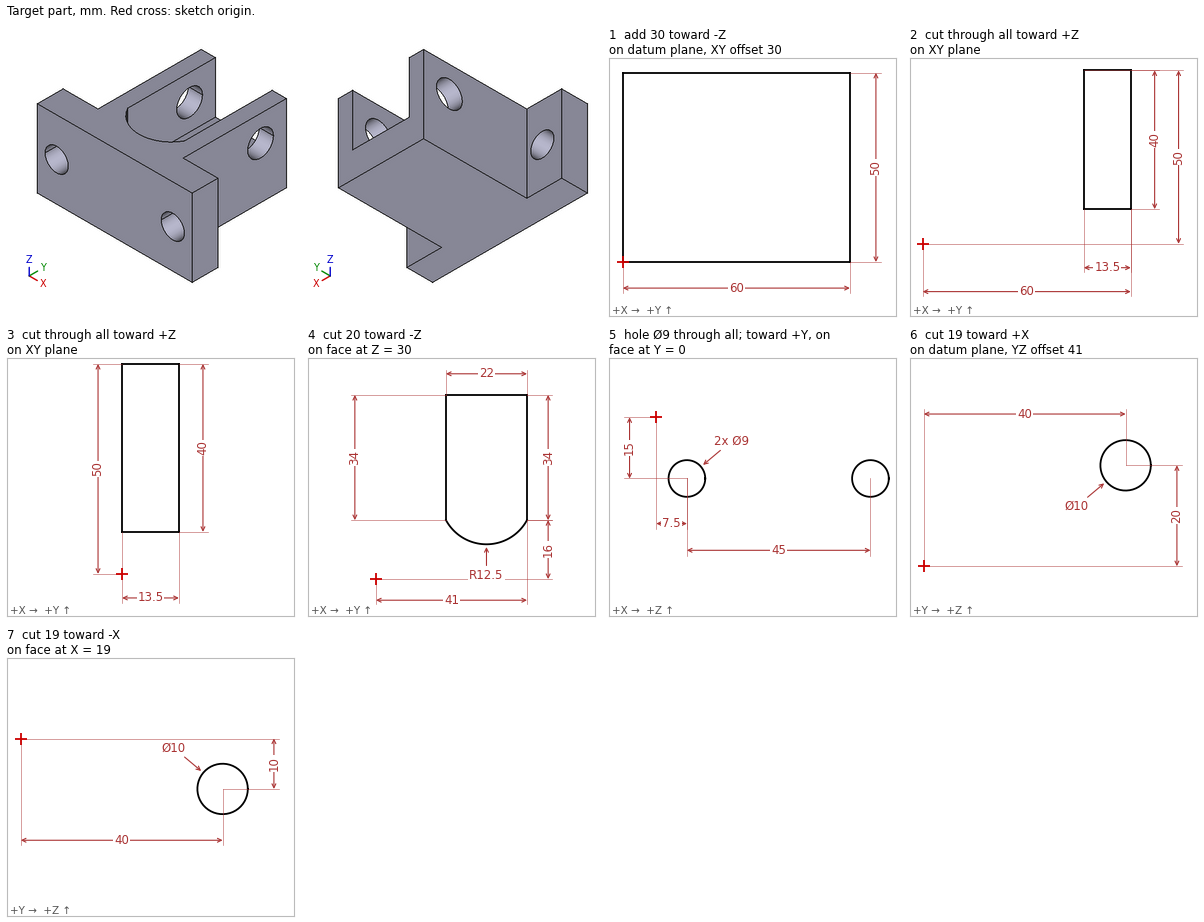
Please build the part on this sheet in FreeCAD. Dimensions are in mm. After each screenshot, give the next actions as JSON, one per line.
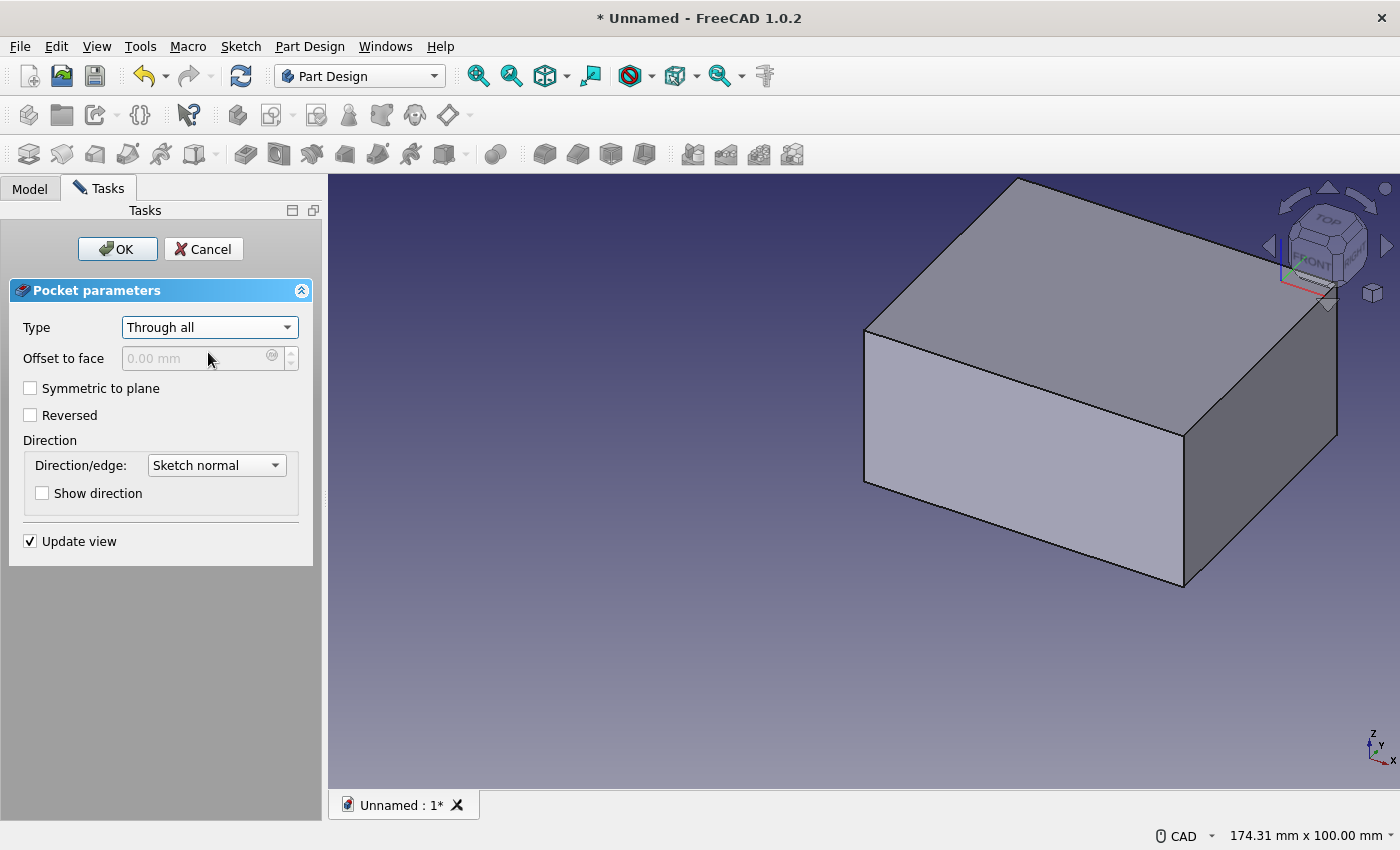
{"action": "left_click", "coordinate": [31, 415]}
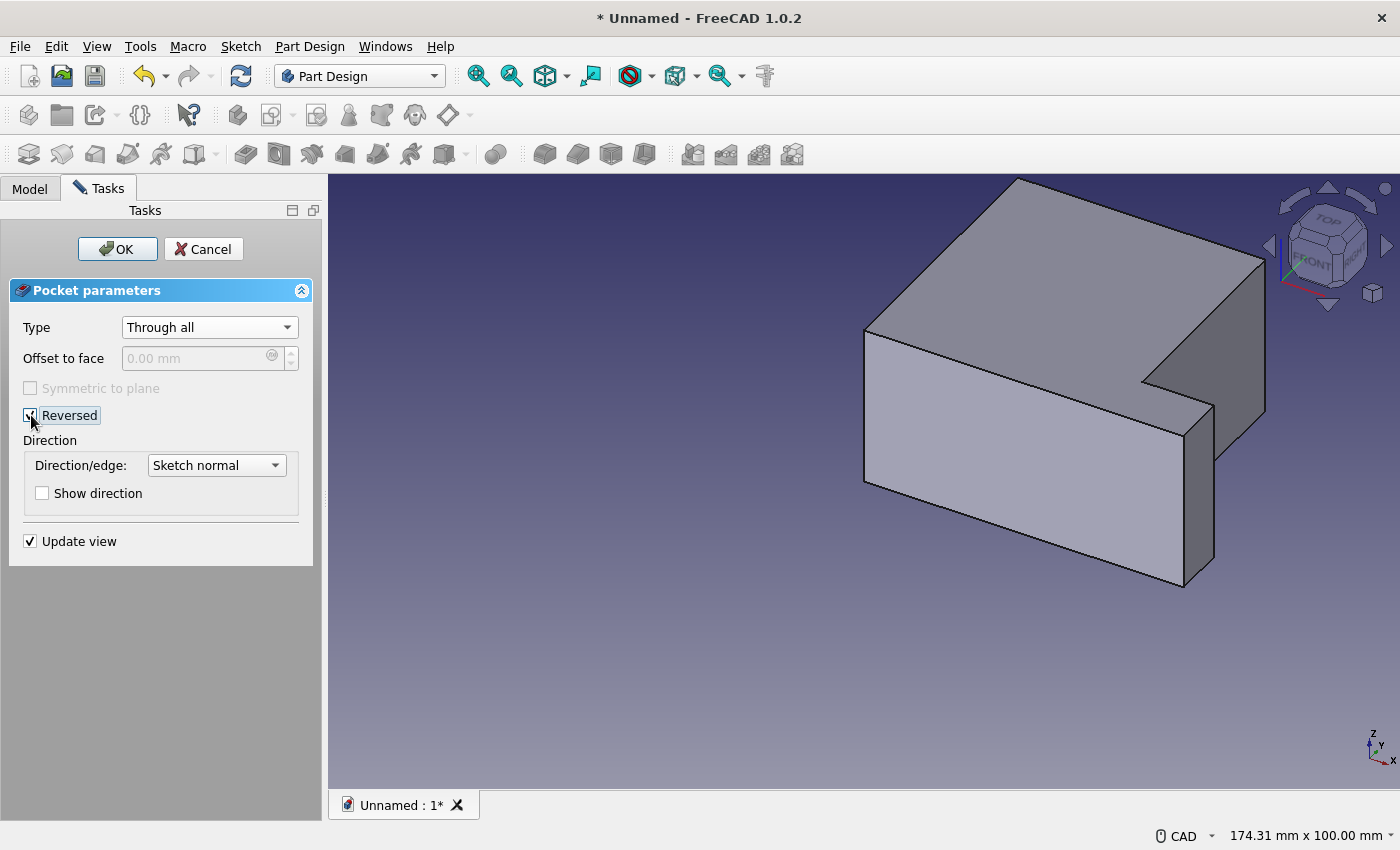
{"action": "left_click", "coordinate": [118, 249]}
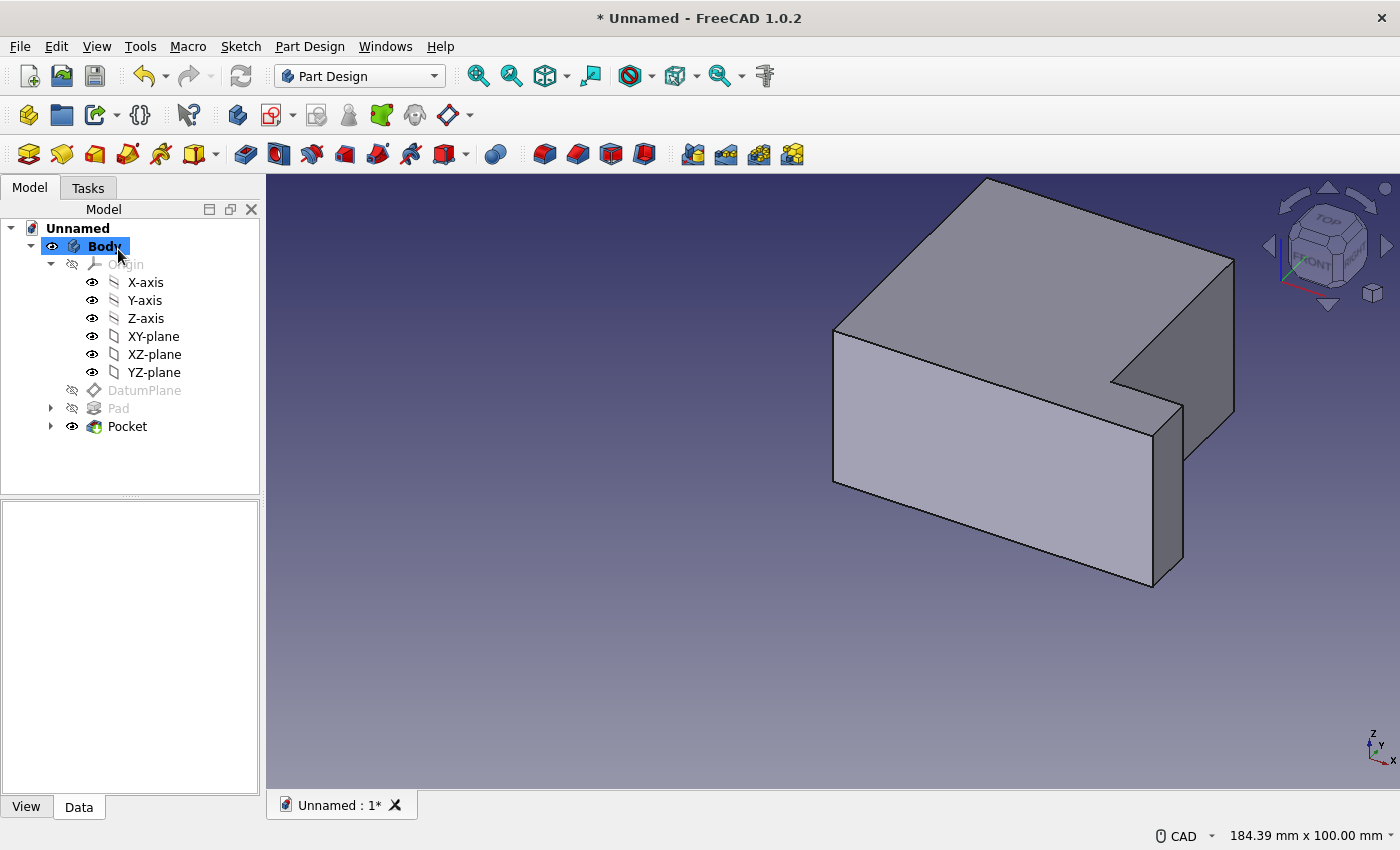
{"action": "left_click", "coordinate": [270, 116]}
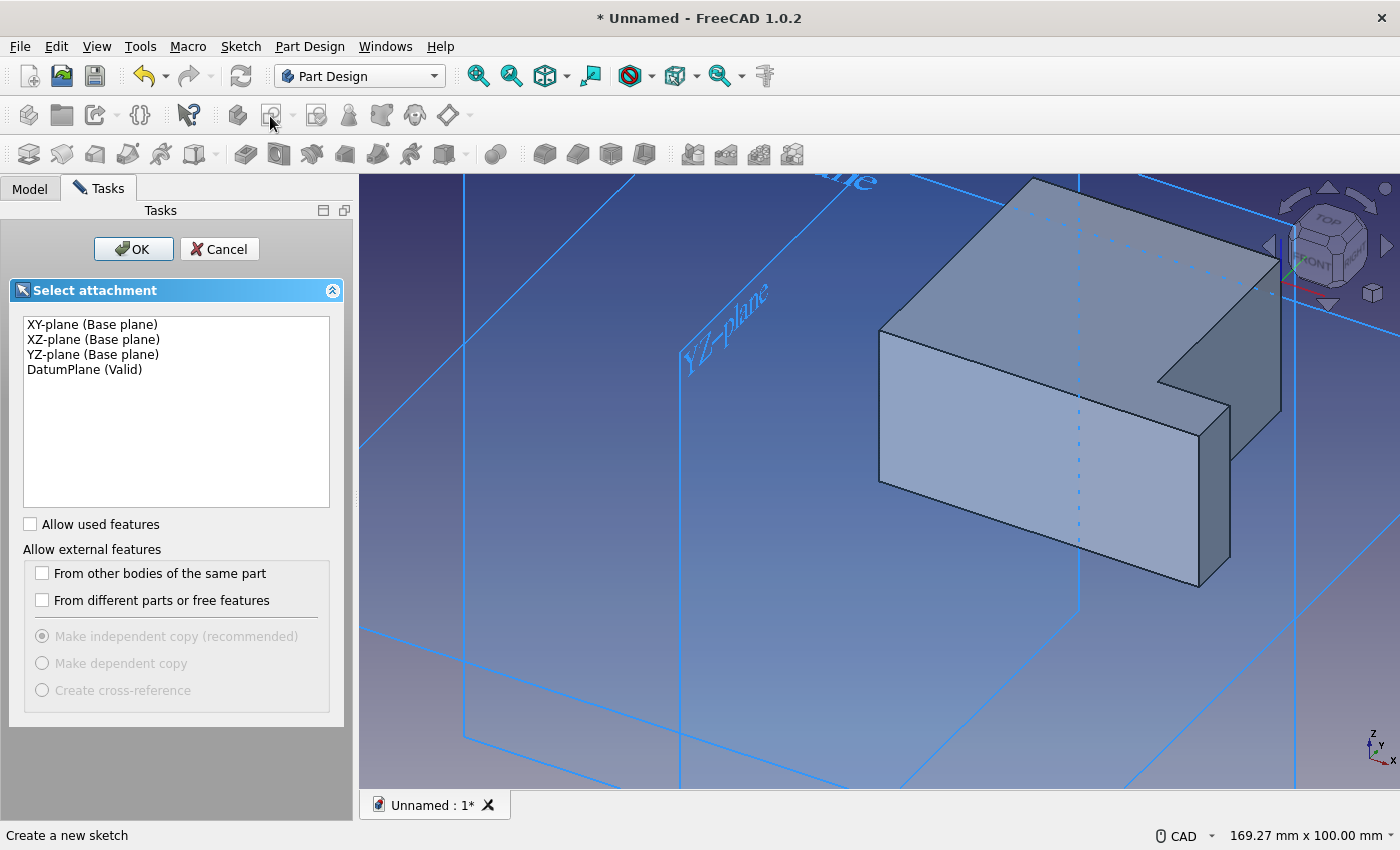
{"action": "left_click", "coordinate": [84, 324]}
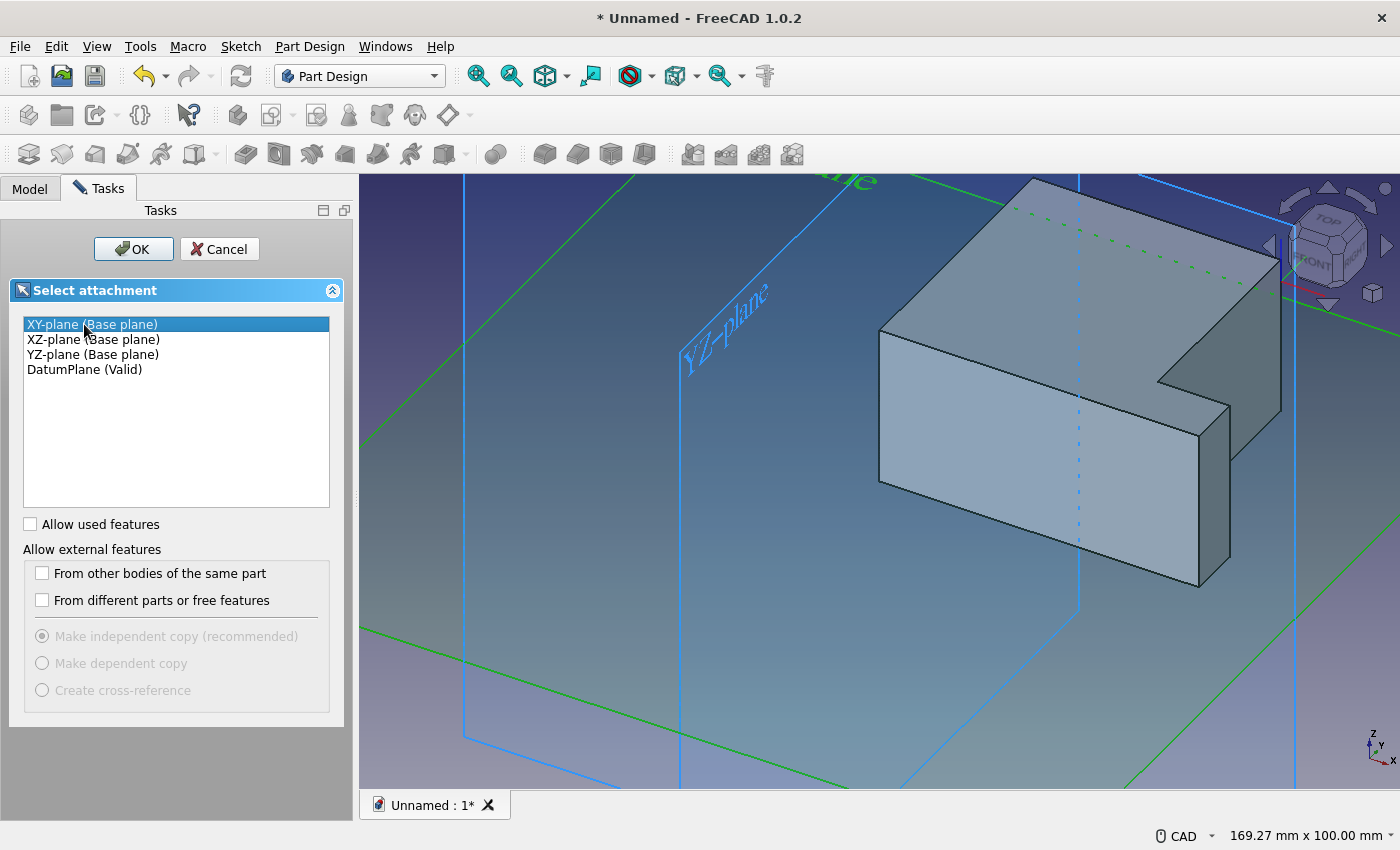
{"action": "left_click", "coordinate": [134, 249]}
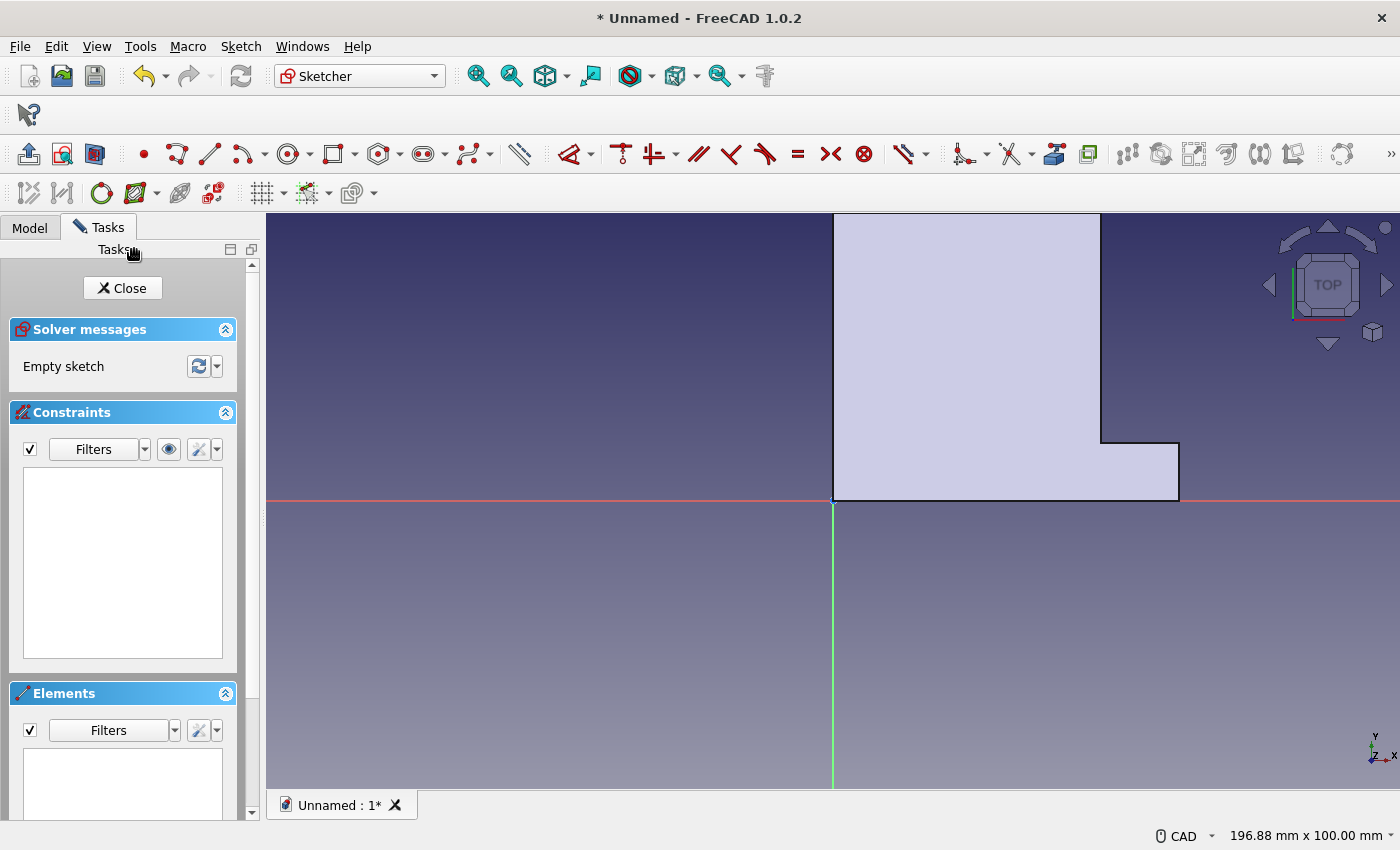
{"action": "key", "text": "q s"}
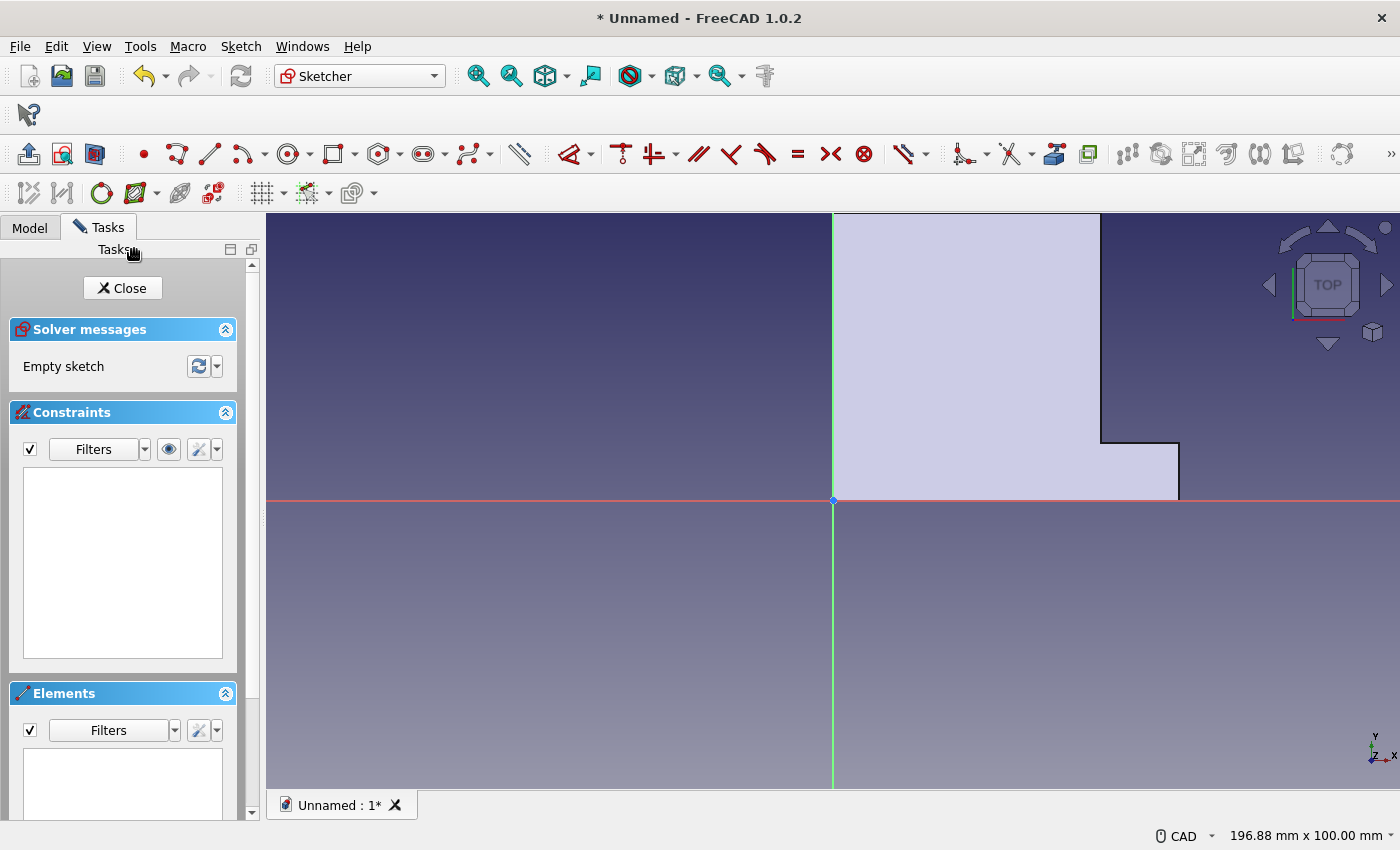
{"action": "scroll", "coordinate": [294, 761], "scroll_direction": "down", "scroll_amount": 1}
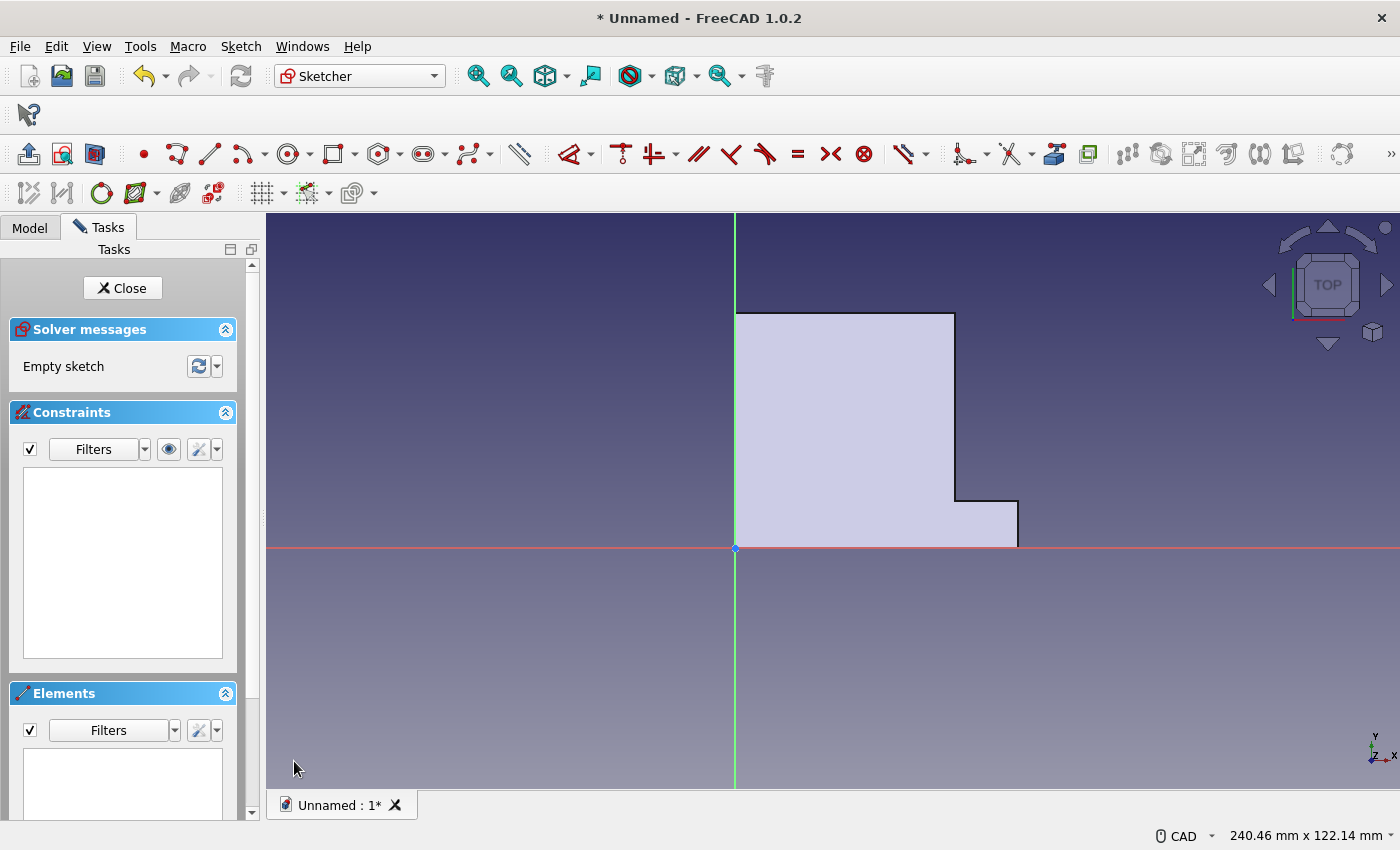
{"action": "scroll", "coordinate": [772, 287], "scroll_direction": "up", "scroll_amount": 2}